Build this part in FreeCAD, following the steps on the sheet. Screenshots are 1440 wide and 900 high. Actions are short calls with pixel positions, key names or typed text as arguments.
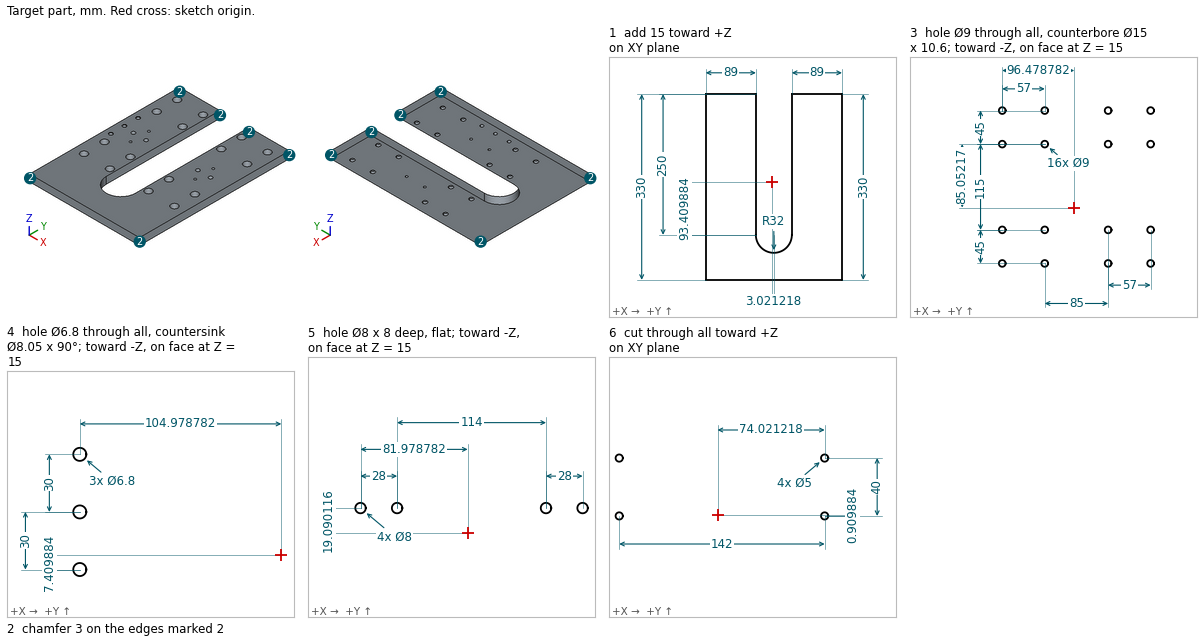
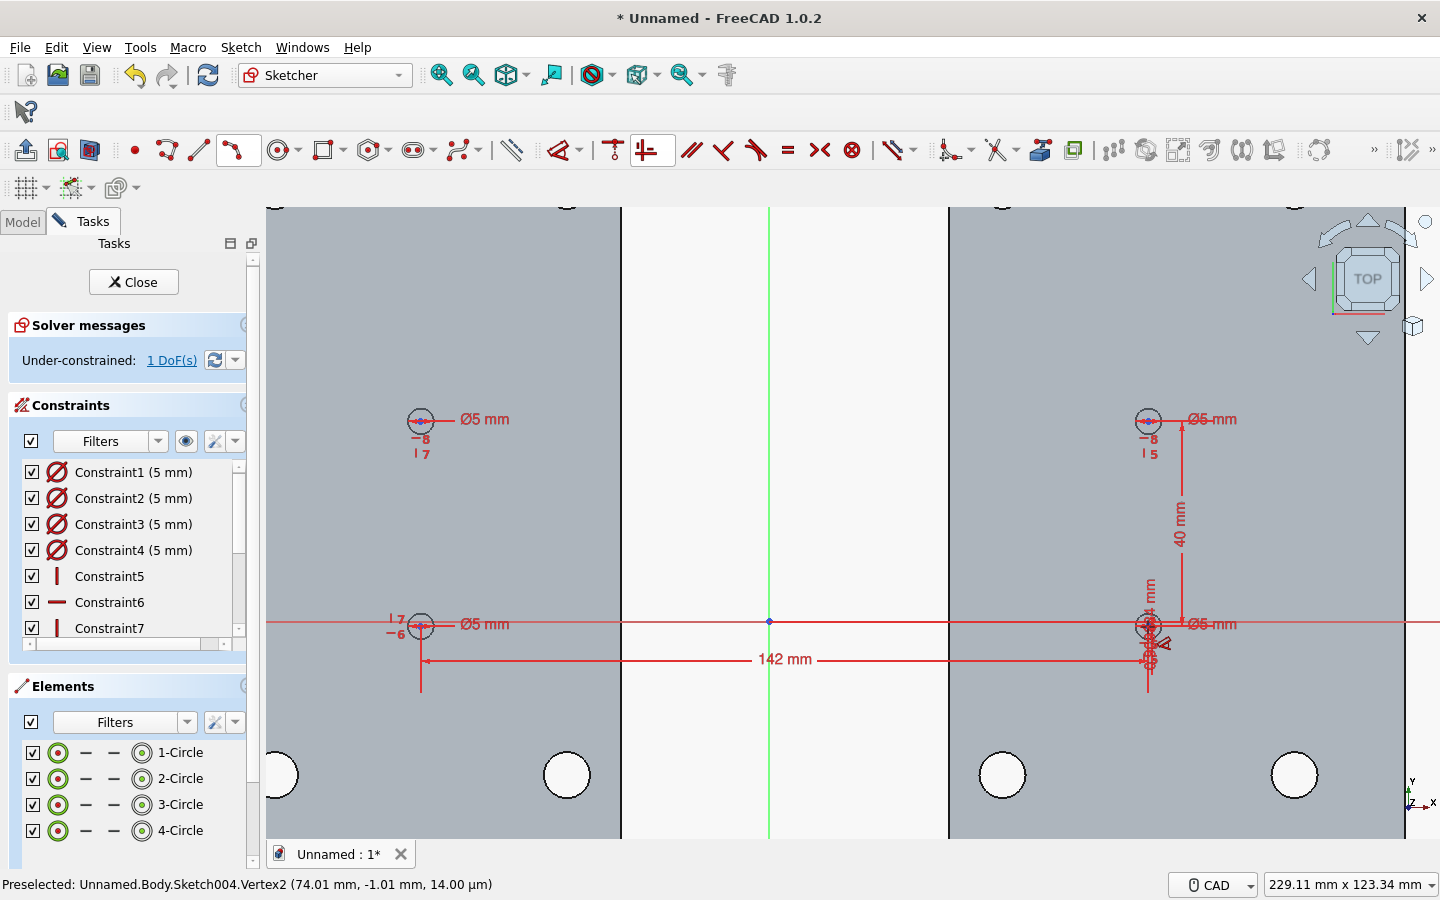
click(1148, 421)
click(959, 387)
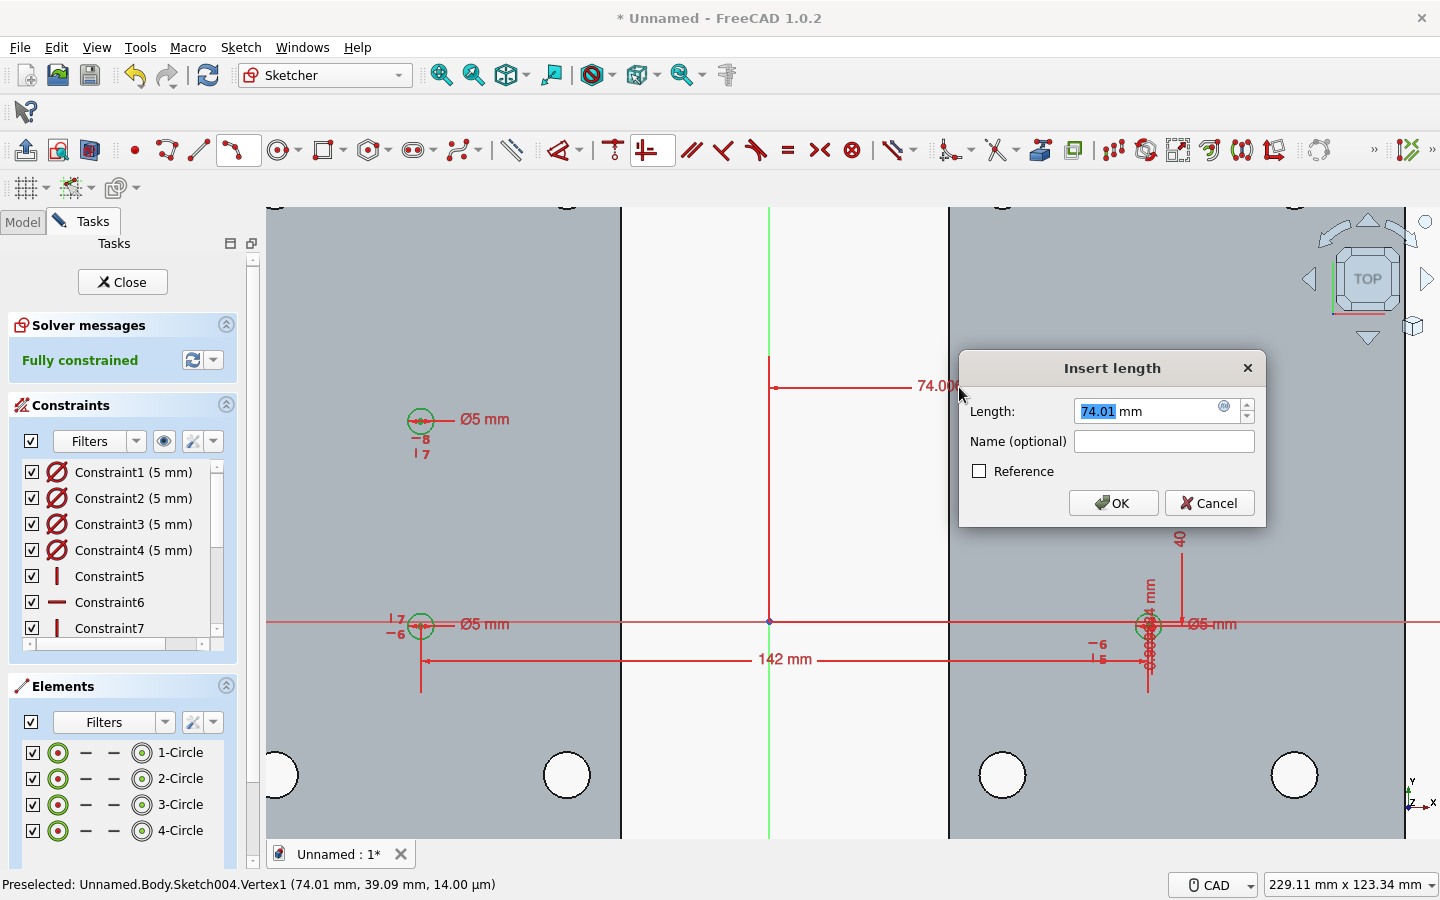
text(74.021218)
key(Return)
key(Escape)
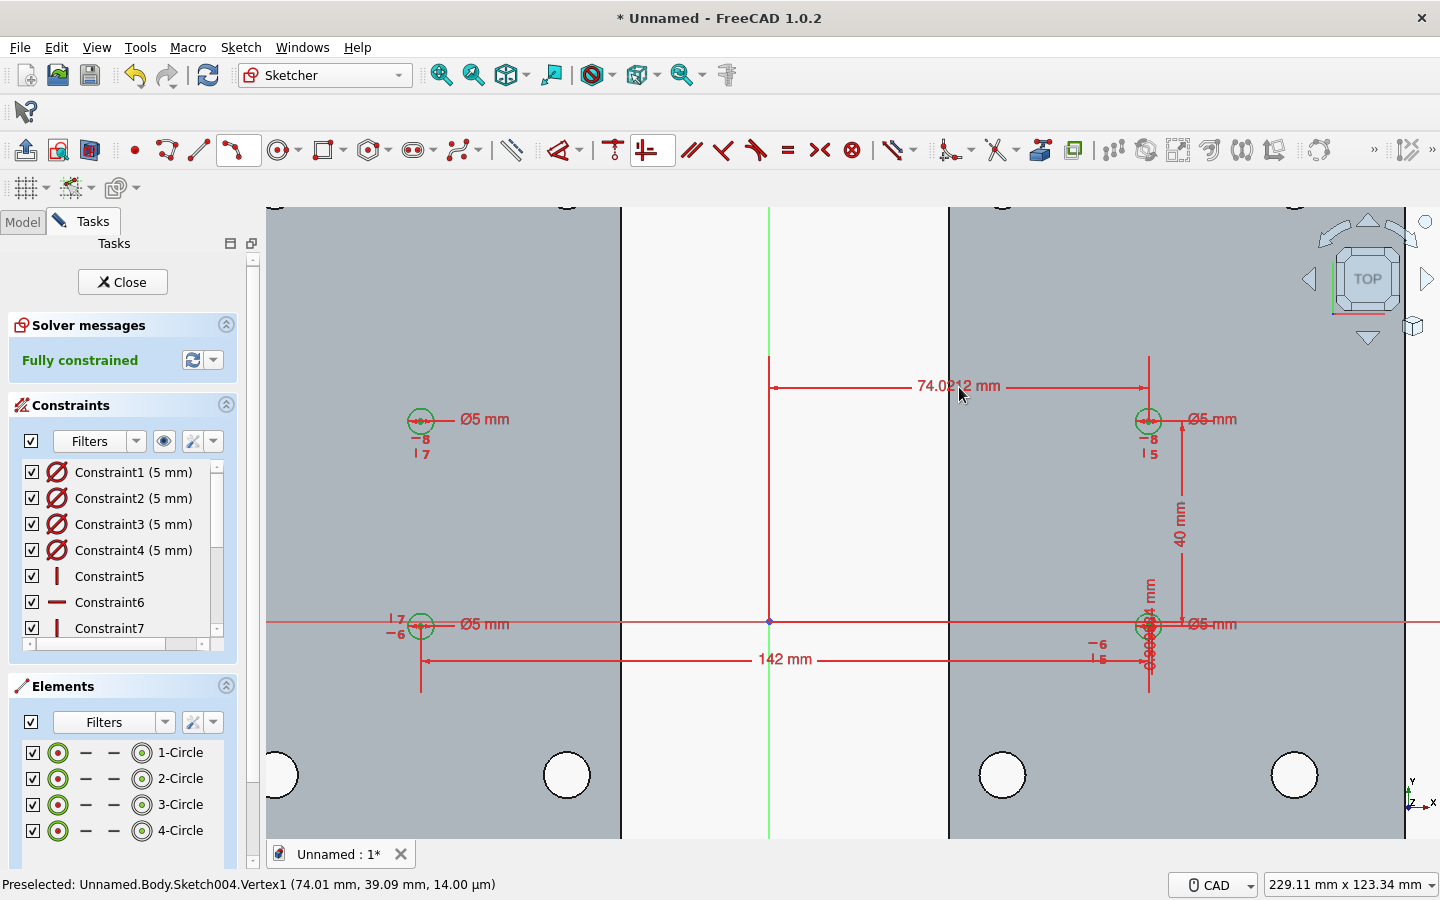
click(123, 282)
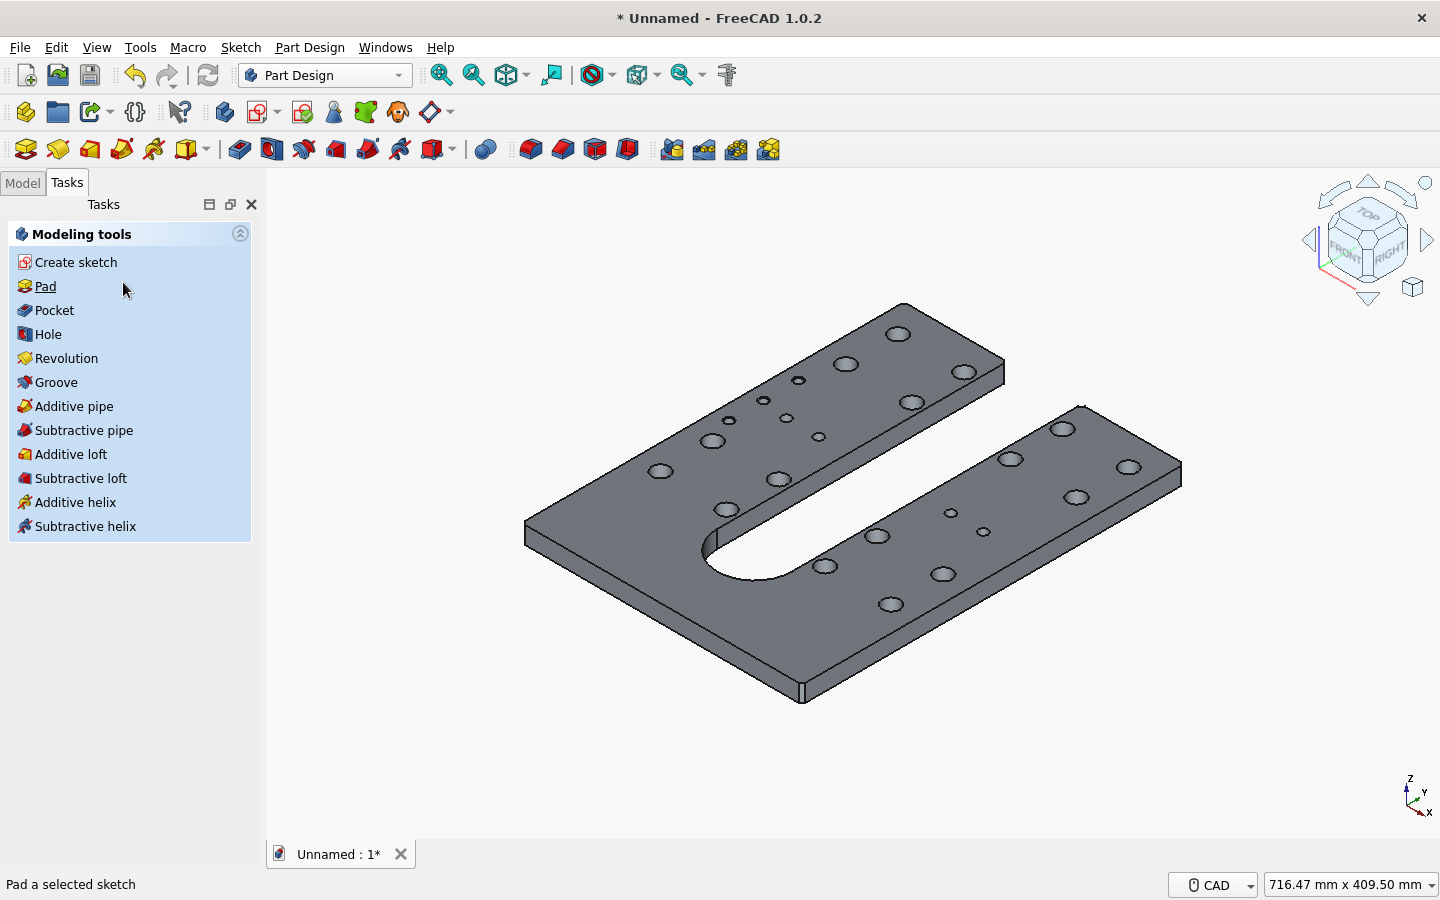
click(240, 150)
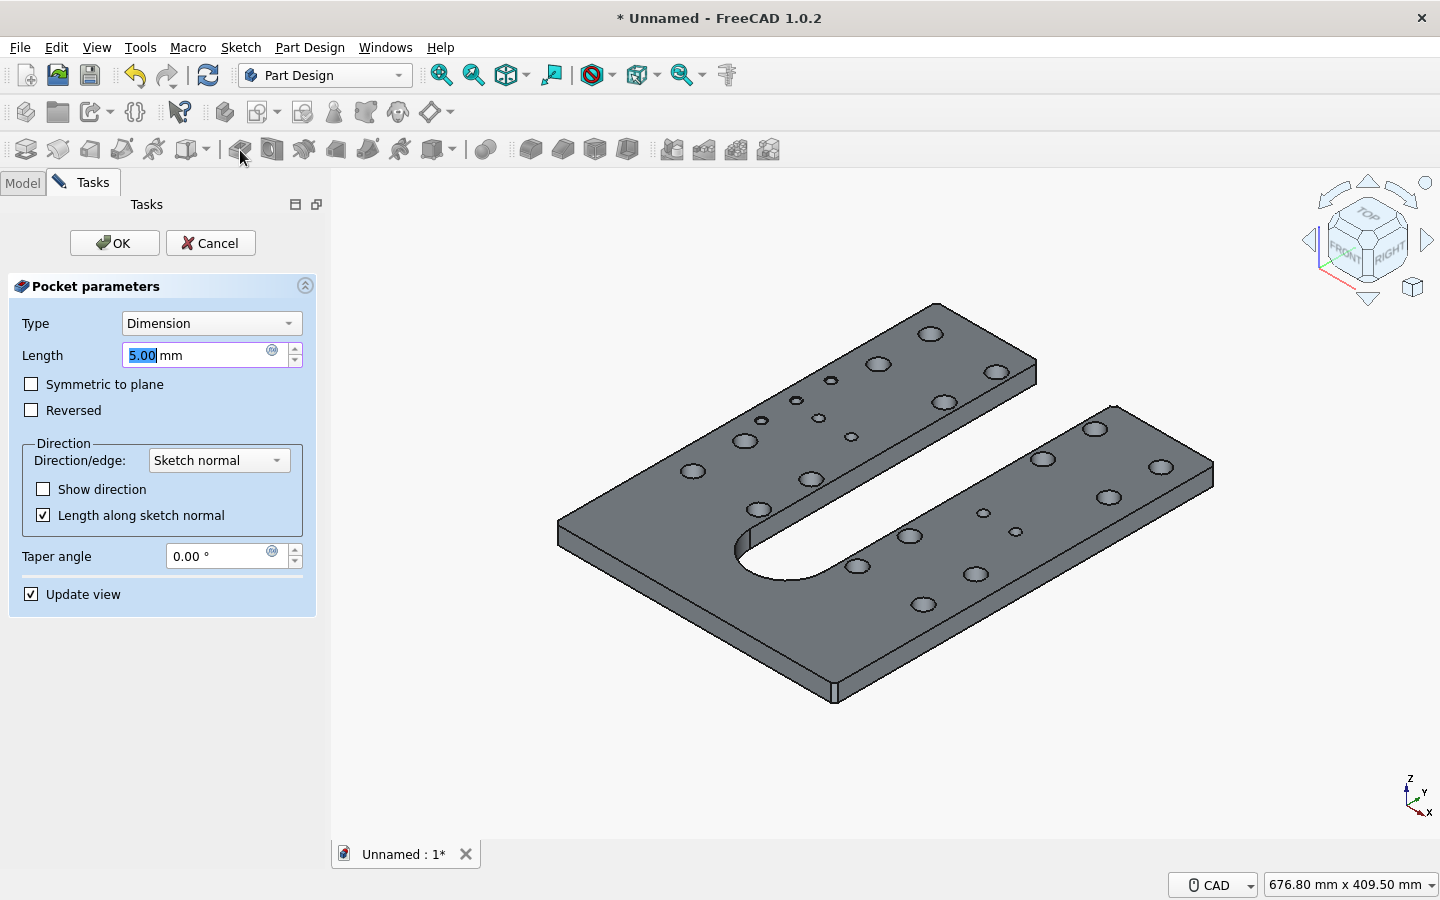
click(212, 324)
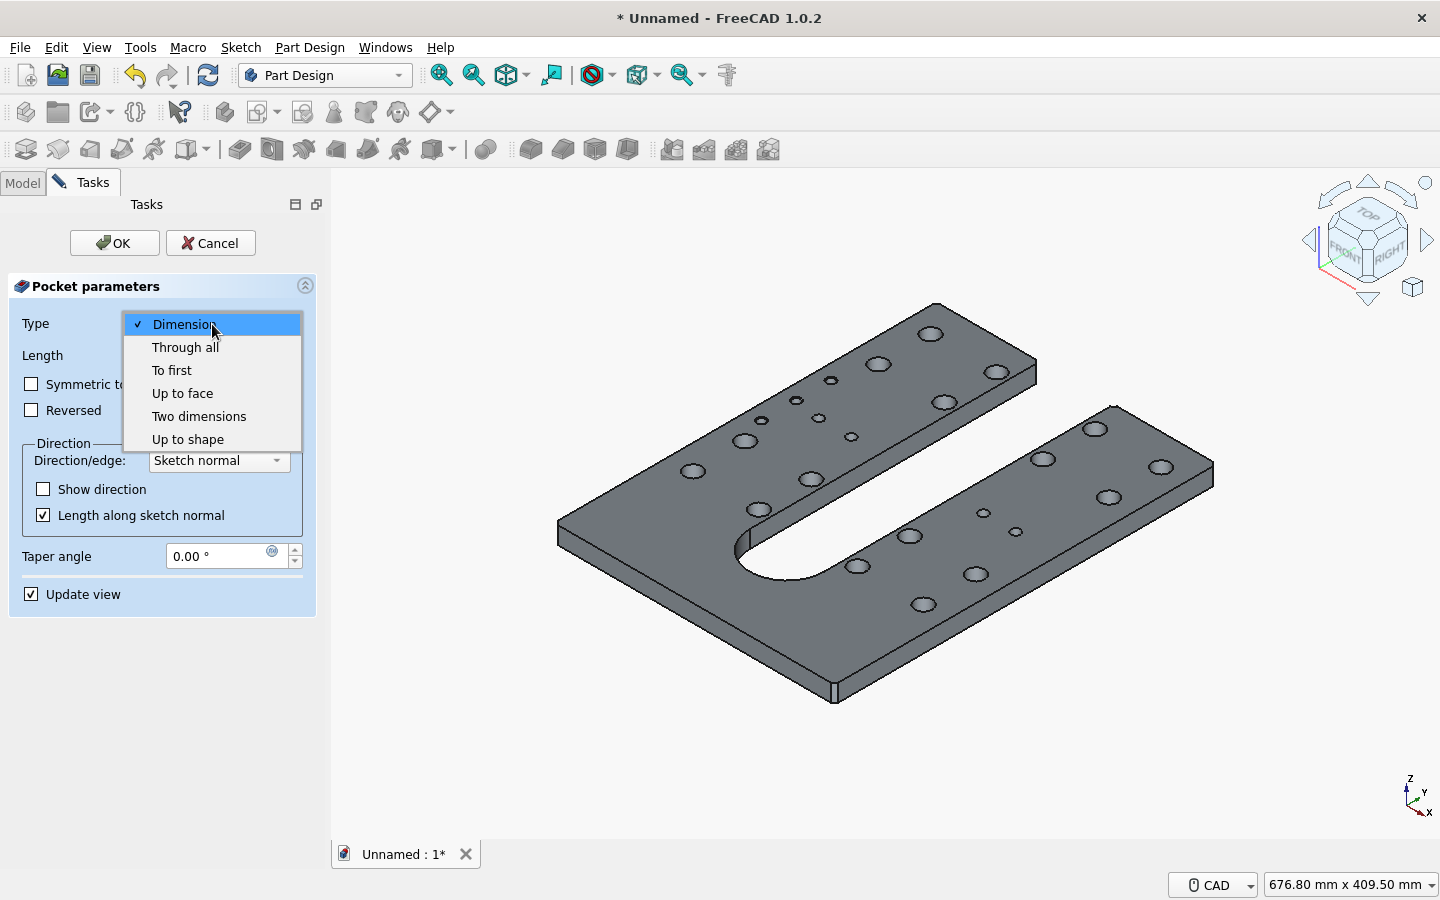
click(212, 348)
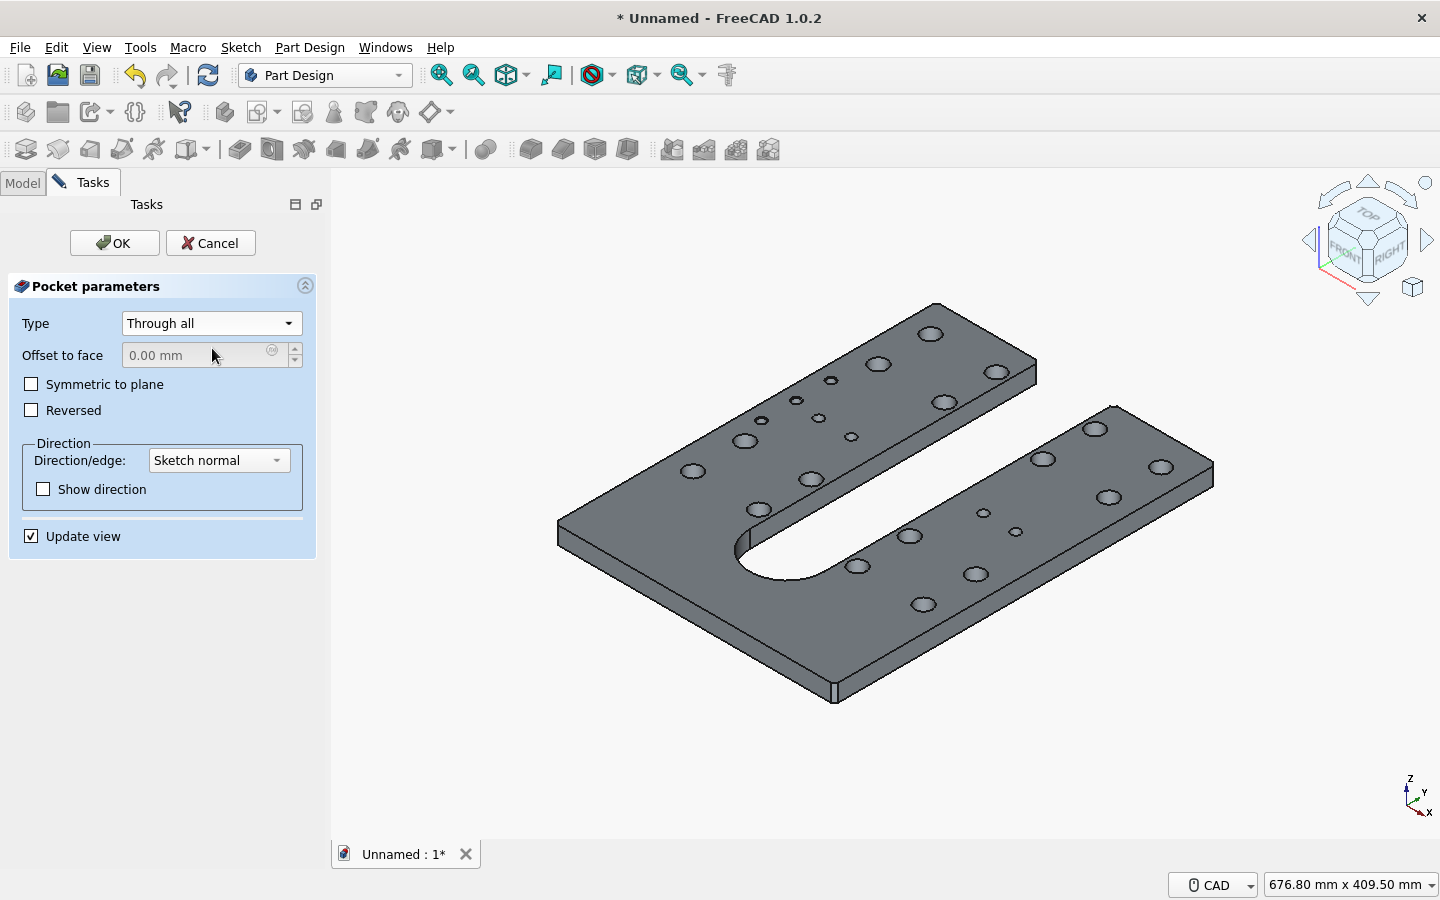
click(30, 410)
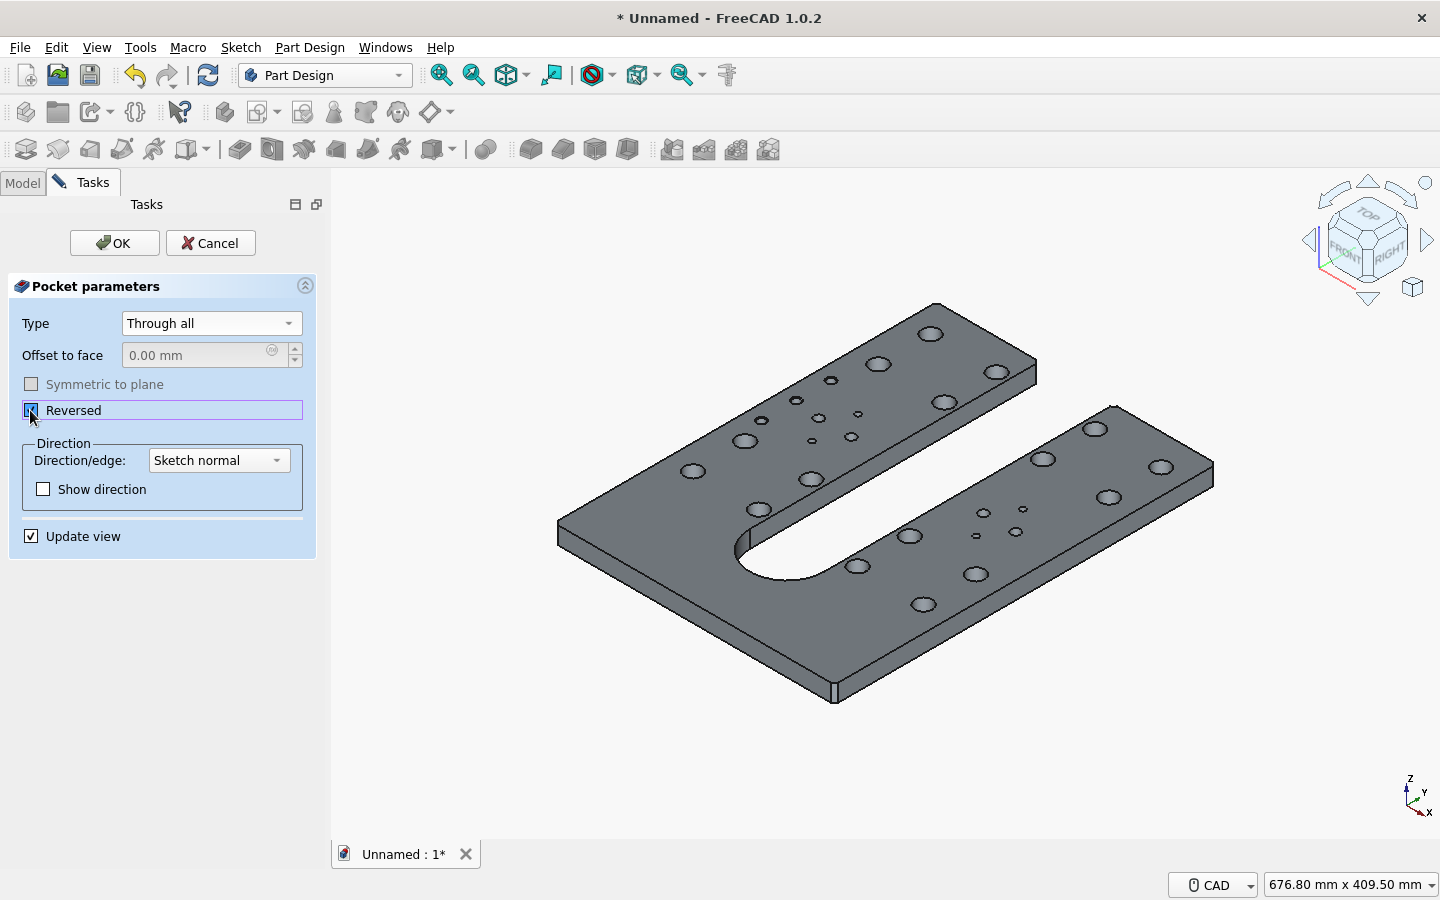
click(115, 243)